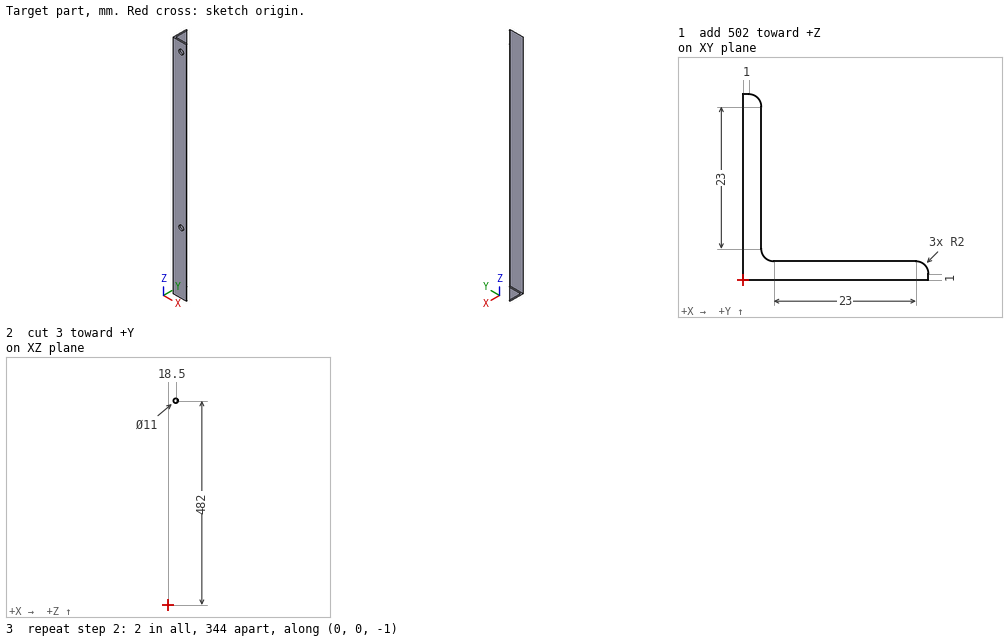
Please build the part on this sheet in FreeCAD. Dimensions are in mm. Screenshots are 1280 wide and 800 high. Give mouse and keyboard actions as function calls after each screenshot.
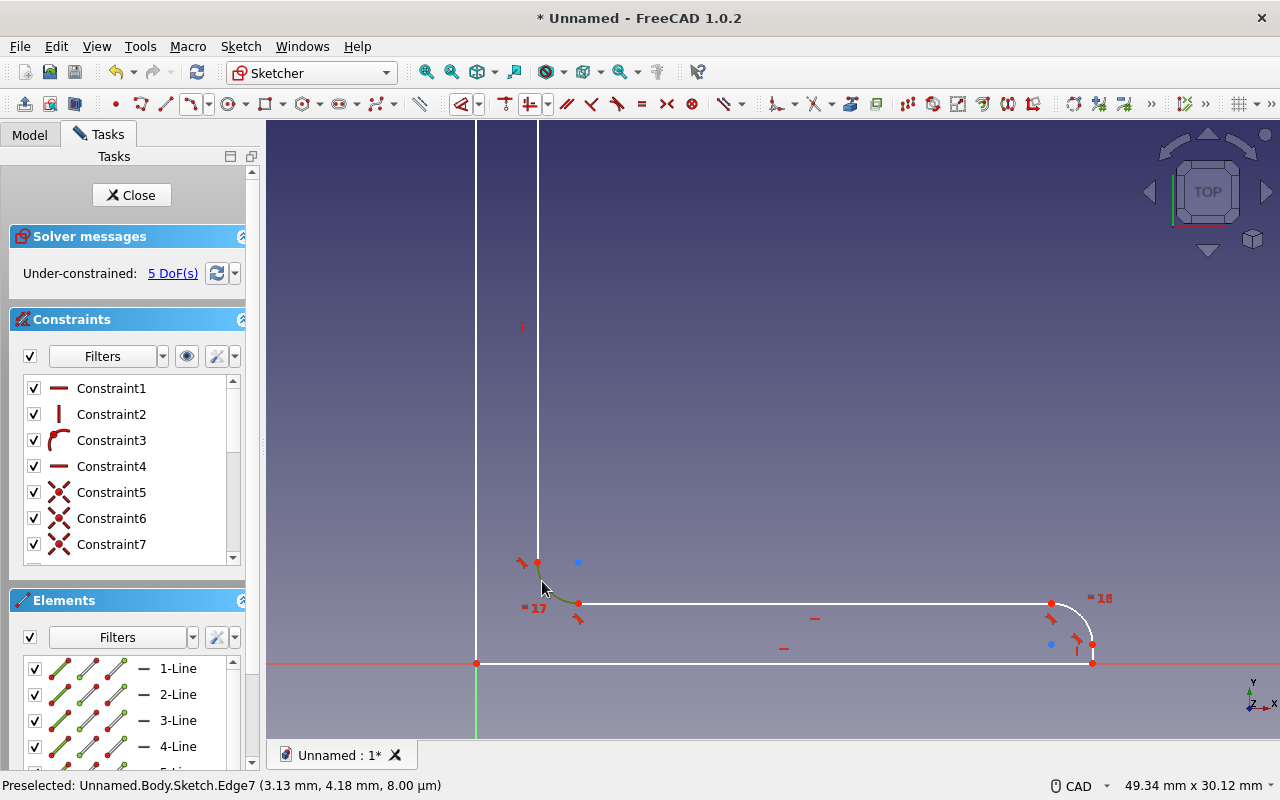
click(478, 104)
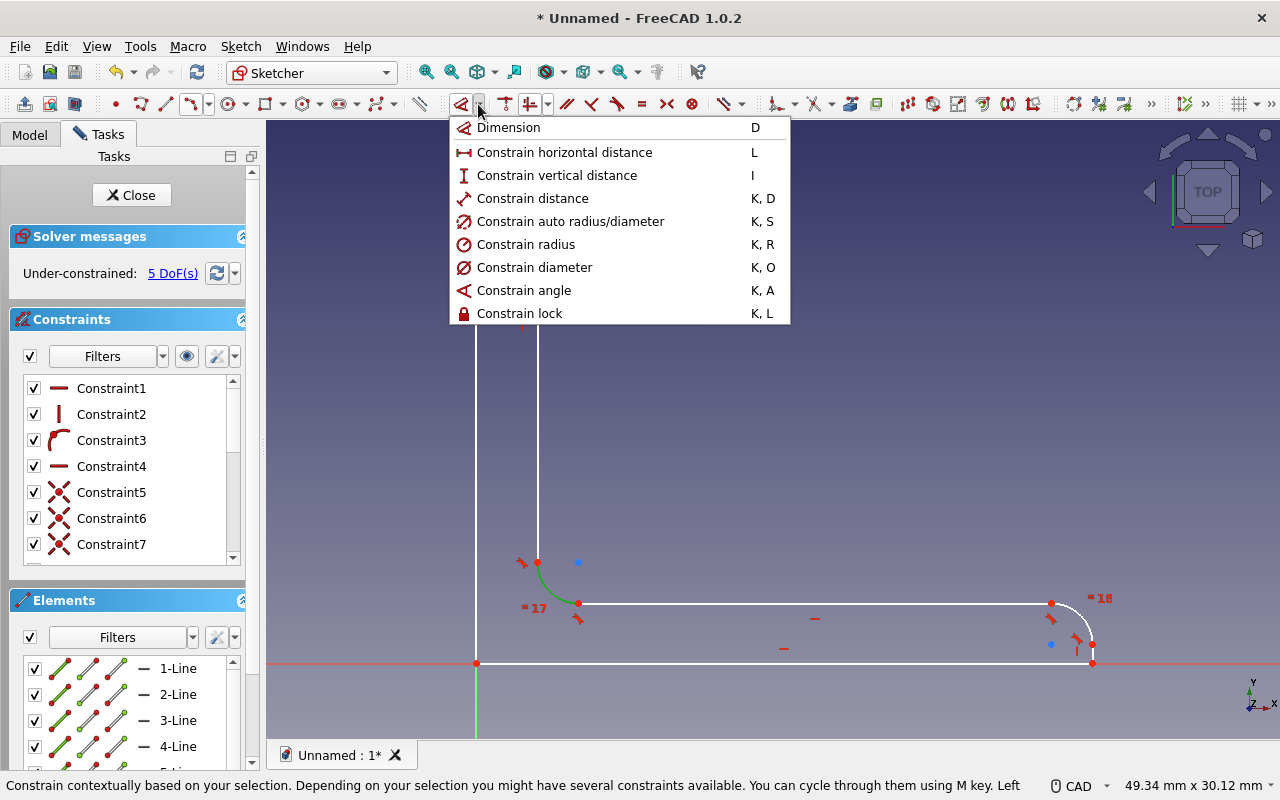
click(620, 244)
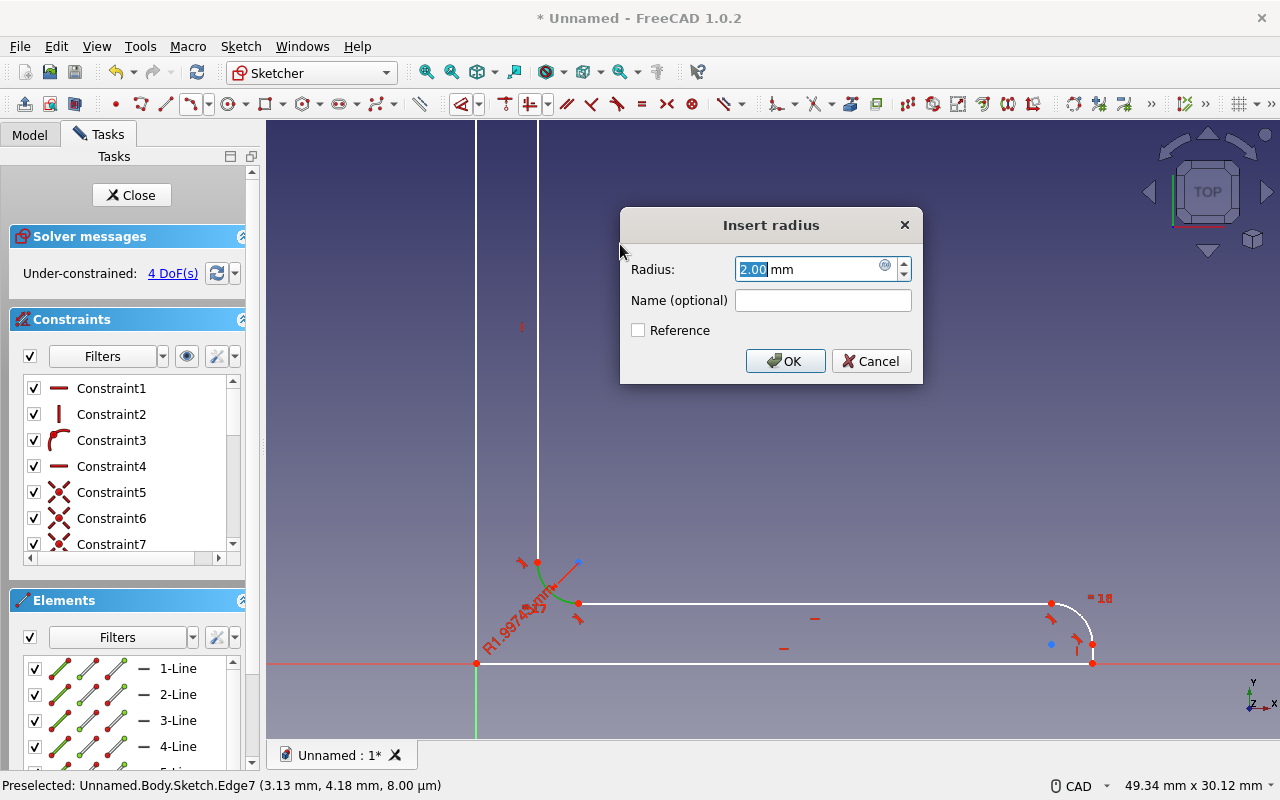
text(2)
key(Return)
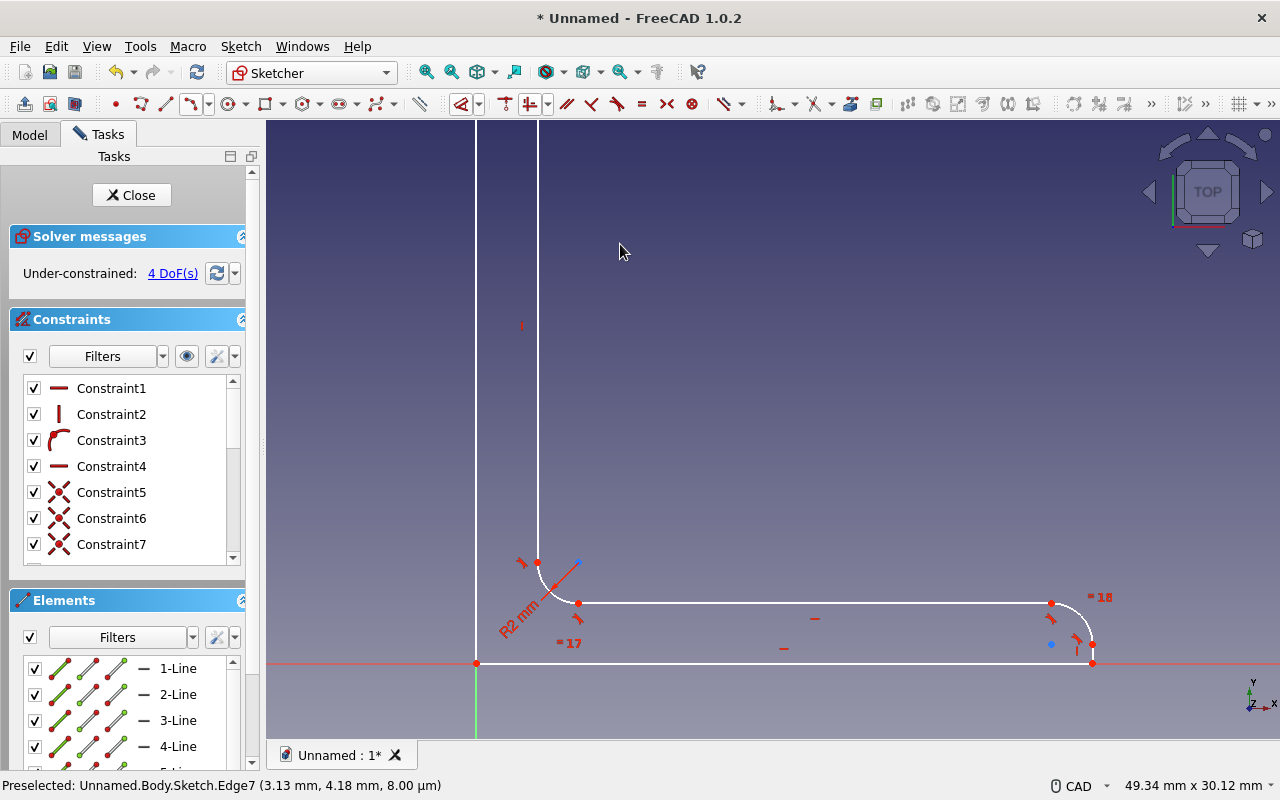
scroll(542, 580, down, 2)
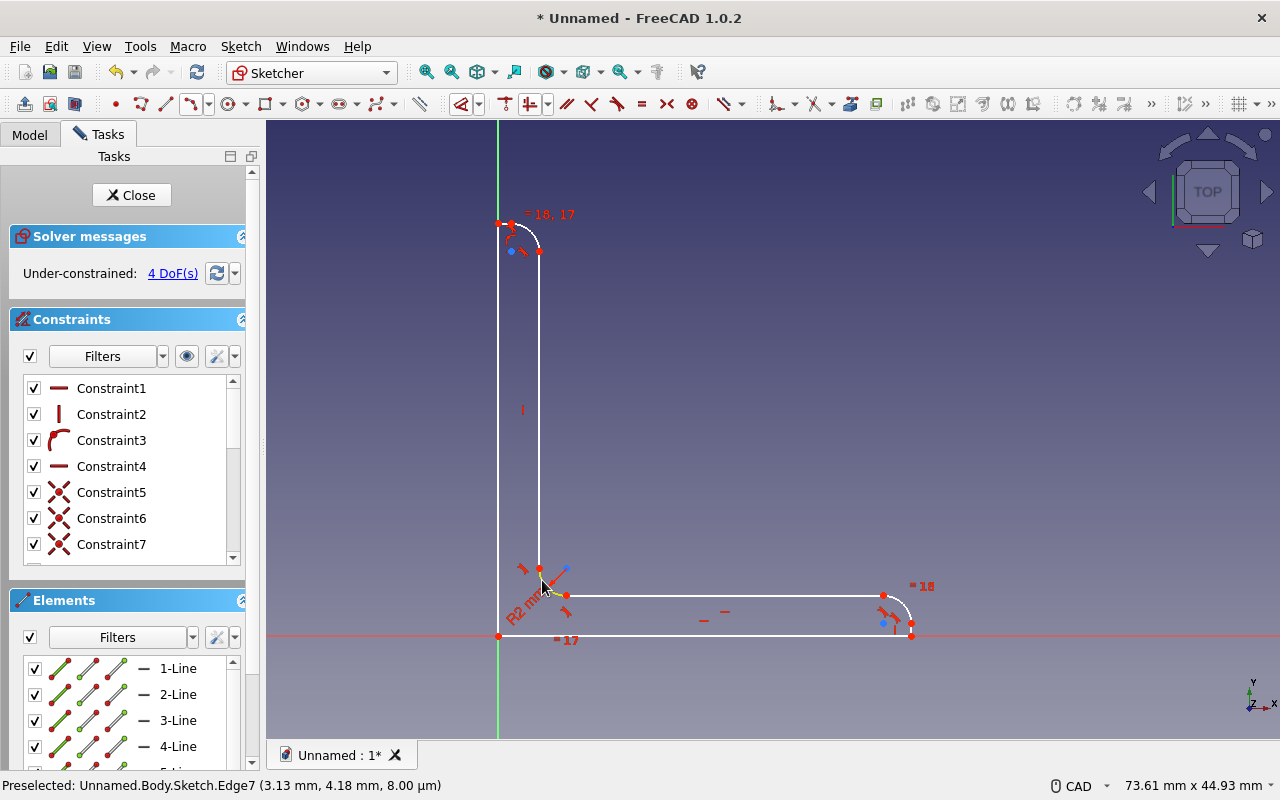
scroll(505, 224, up, 6)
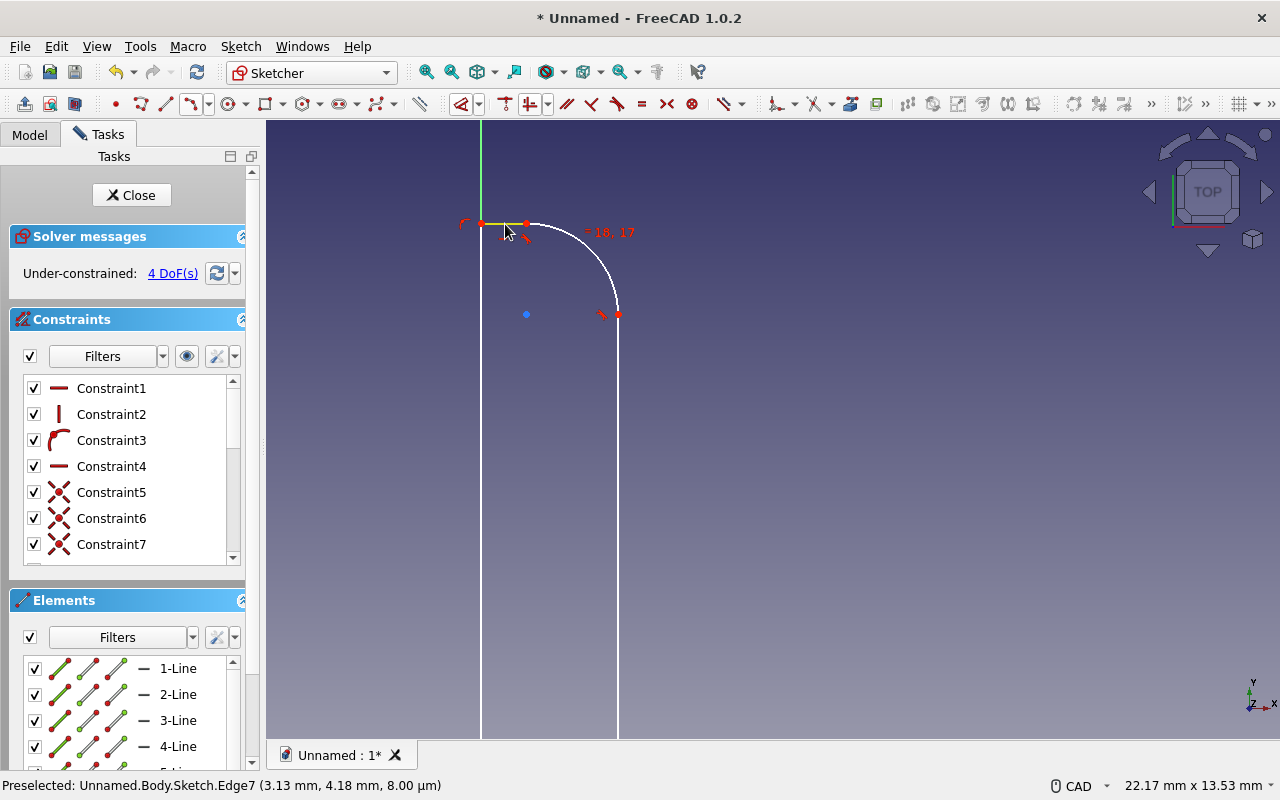
click(504, 224)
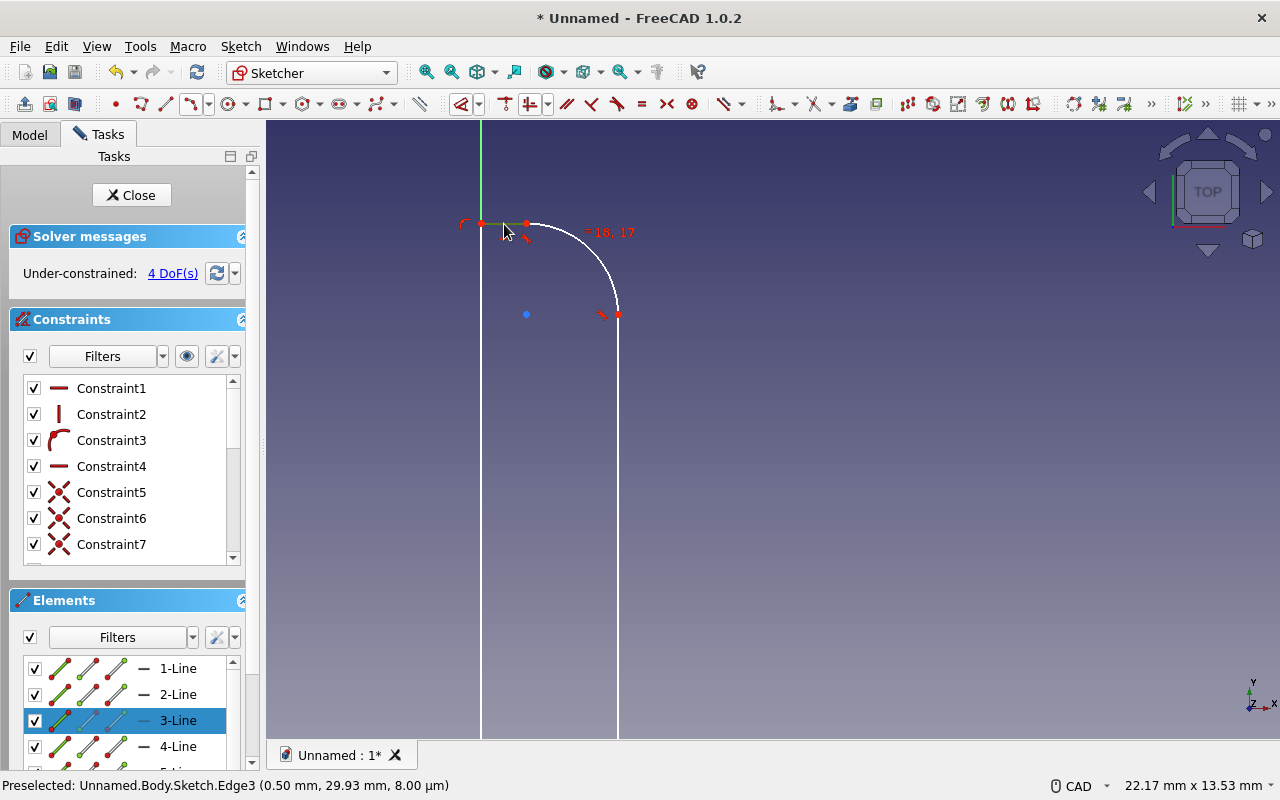
key(l)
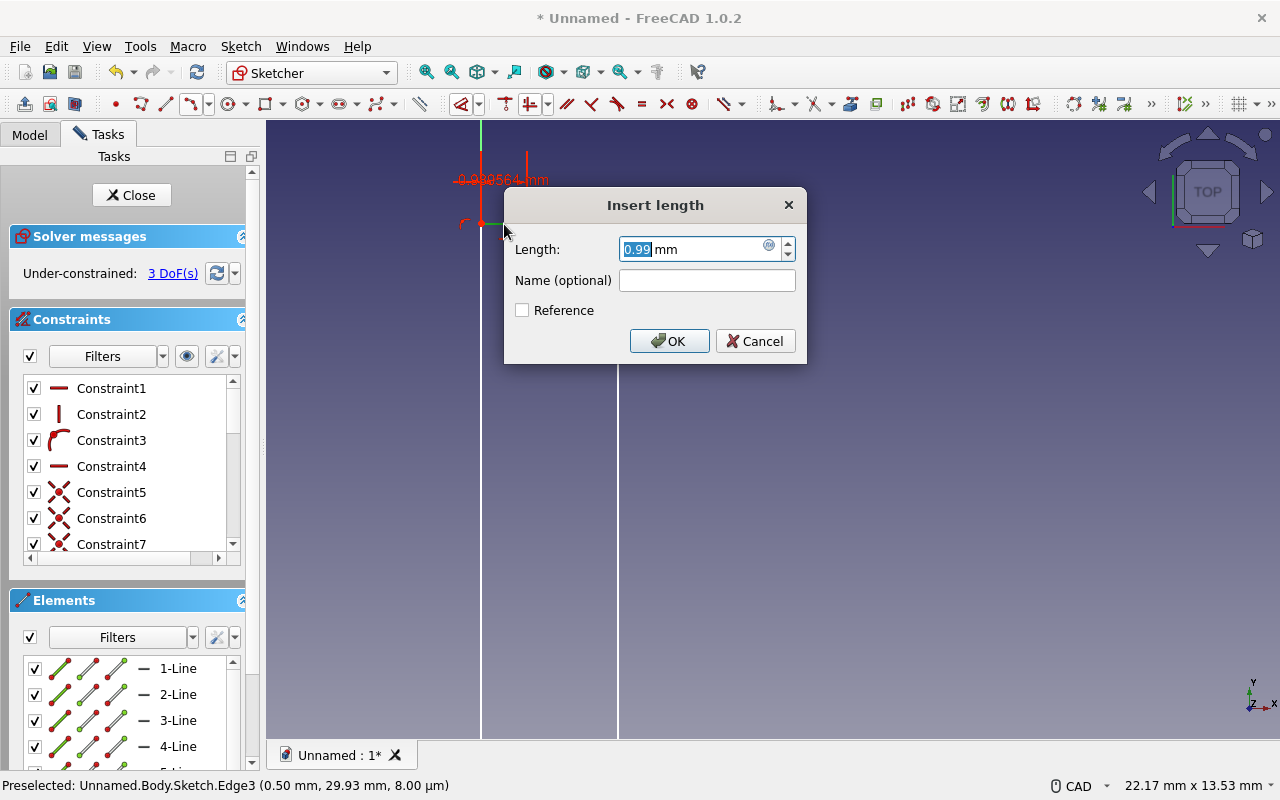
text(1)
key(Return)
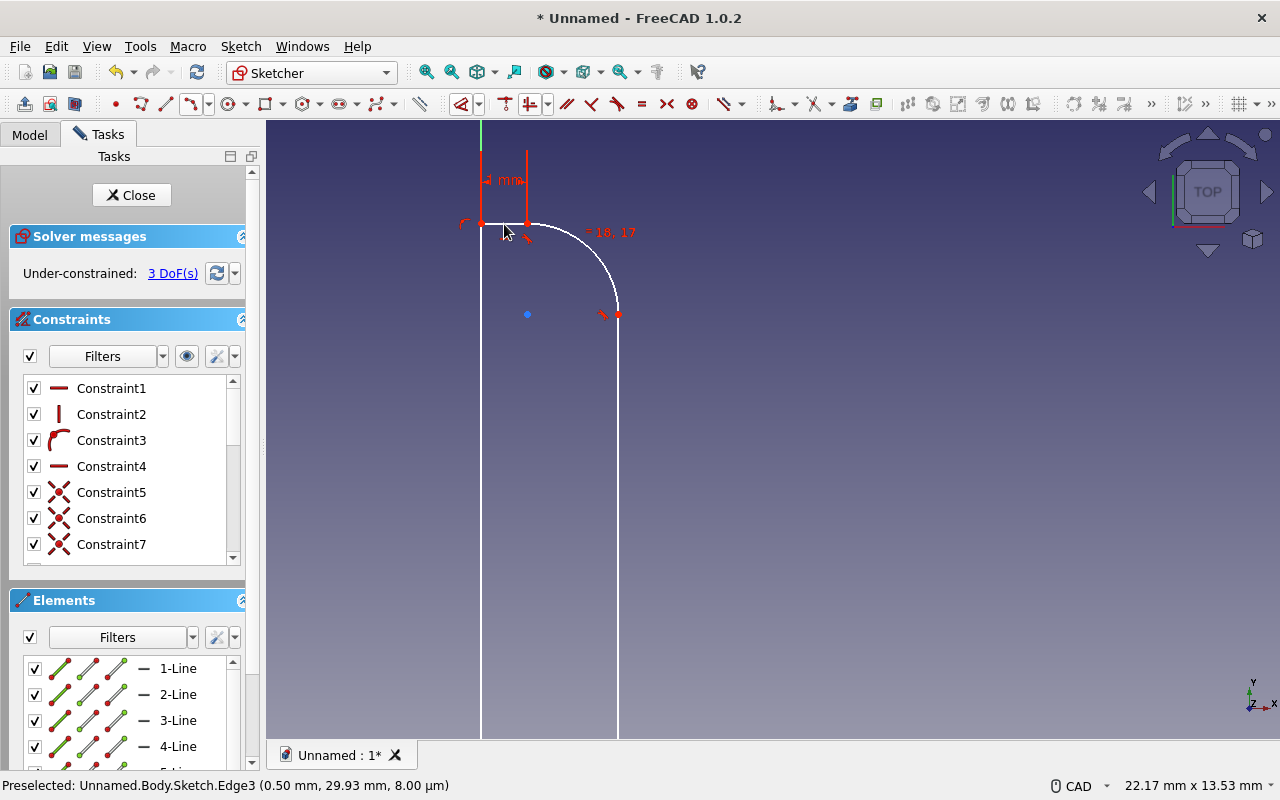
scroll(505, 224, down, 6)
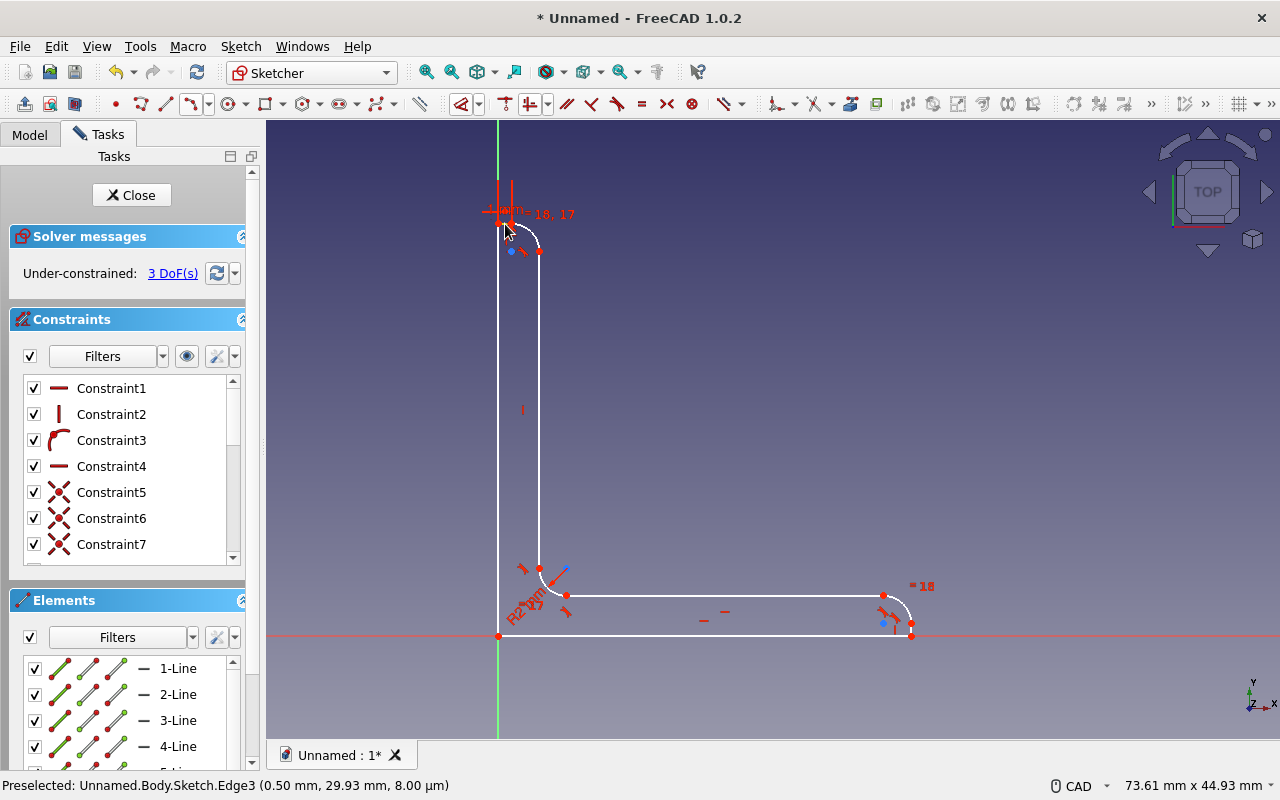
scroll(911, 632, up, 7)